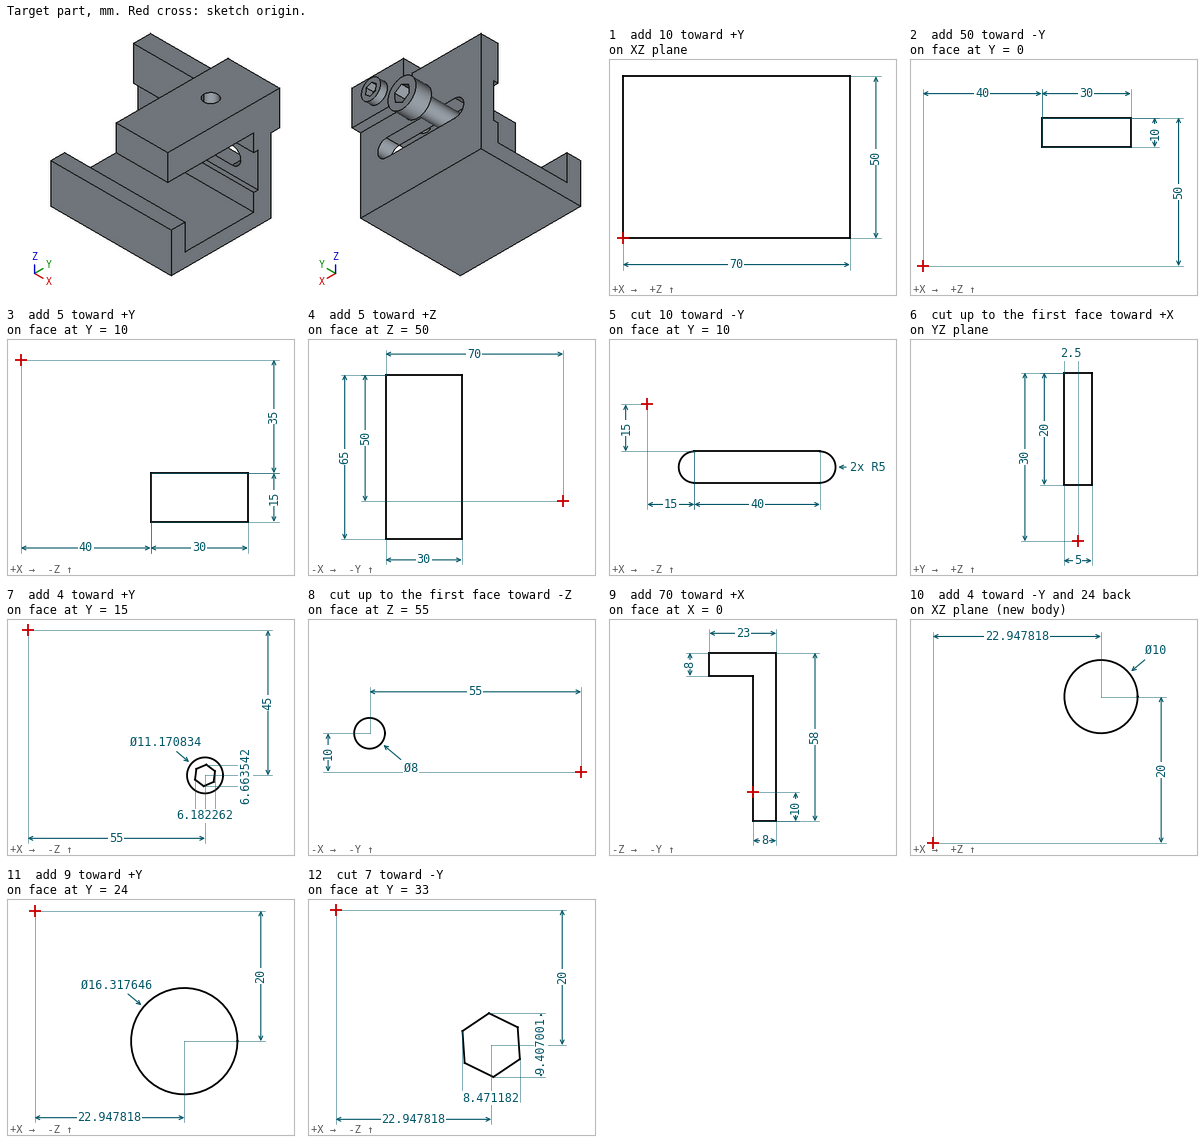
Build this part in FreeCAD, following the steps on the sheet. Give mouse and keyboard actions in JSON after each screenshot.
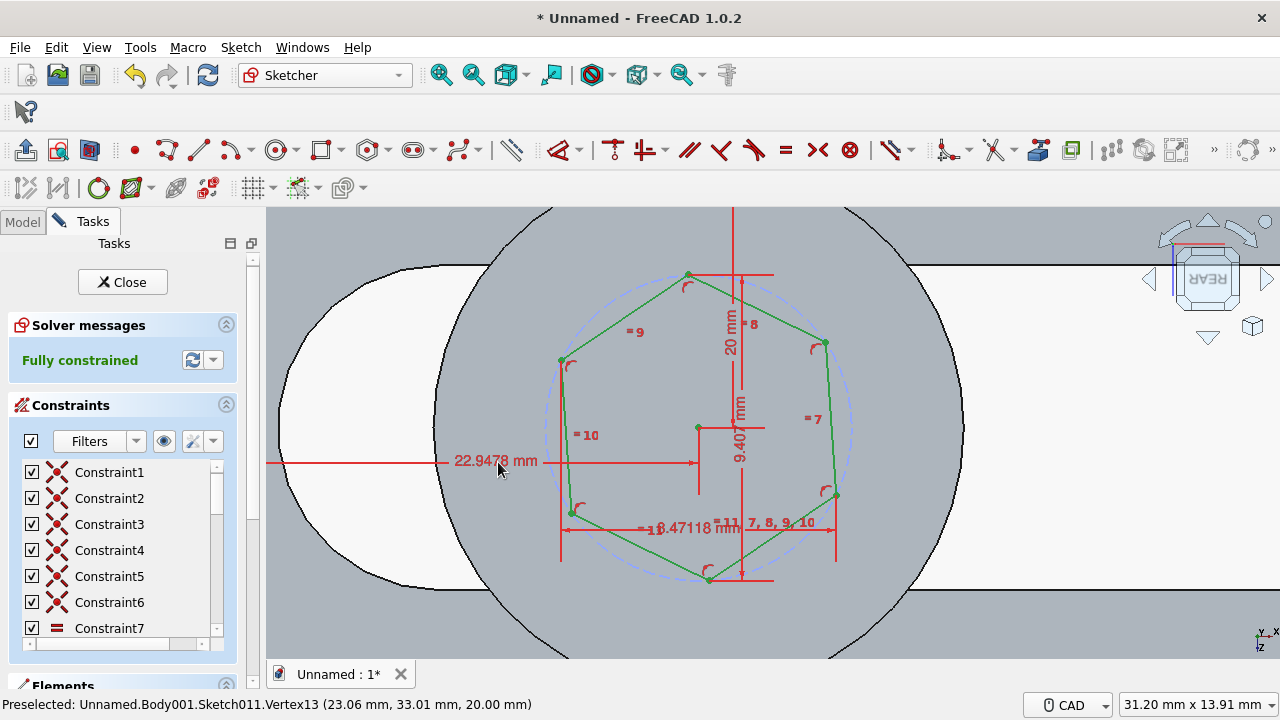
{"action": "left_click", "coordinate": [123, 282]}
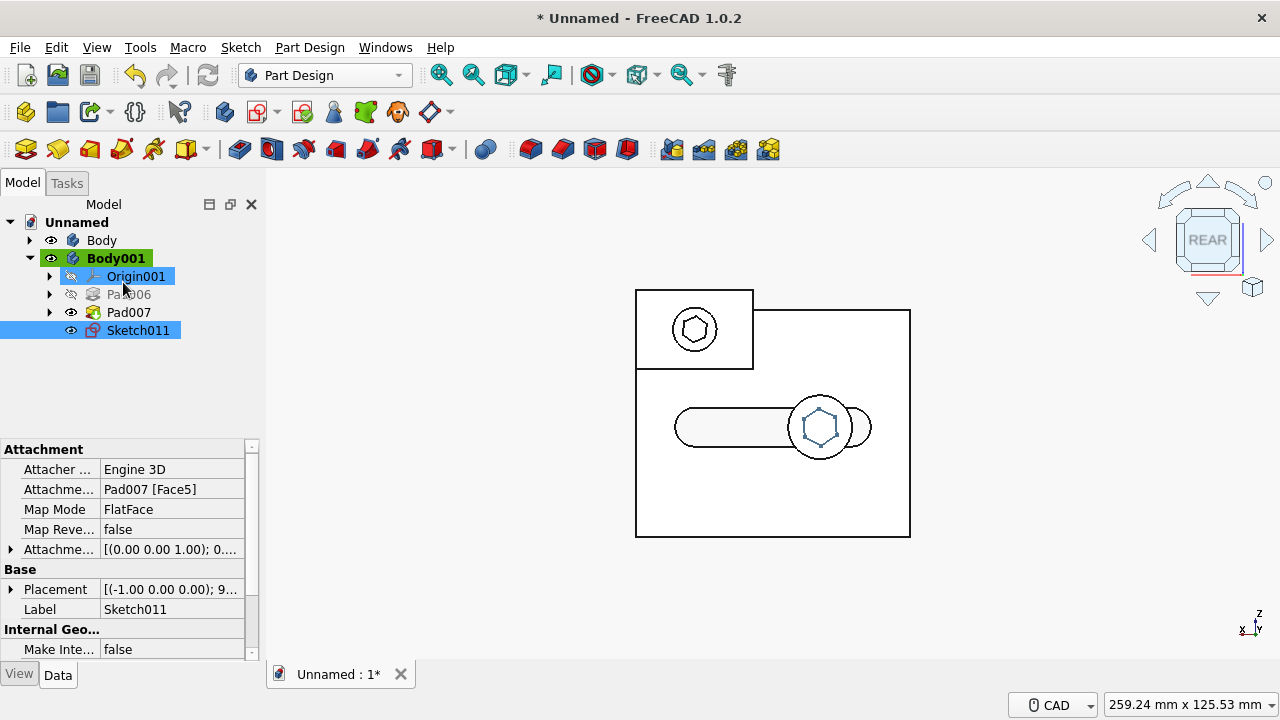
{"action": "left_click", "coordinate": [240, 150]}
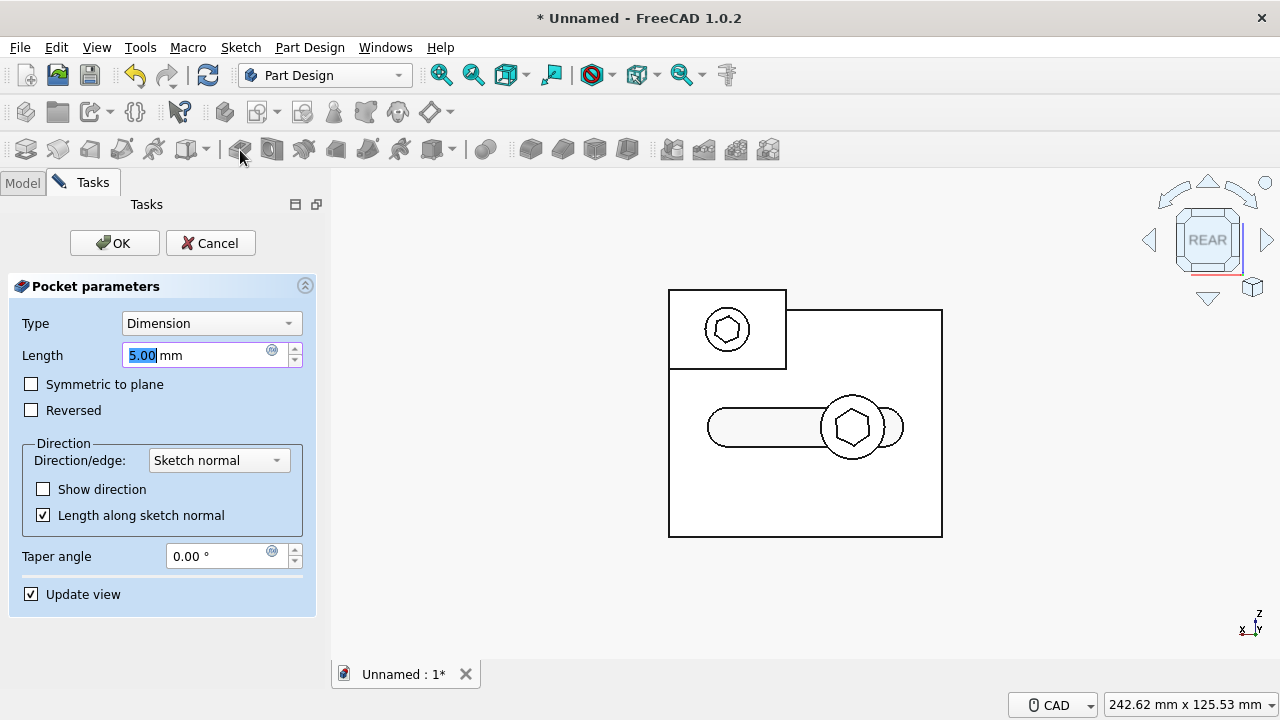
{"action": "type", "text": "7"}
{"action": "key", "text": "Tab"}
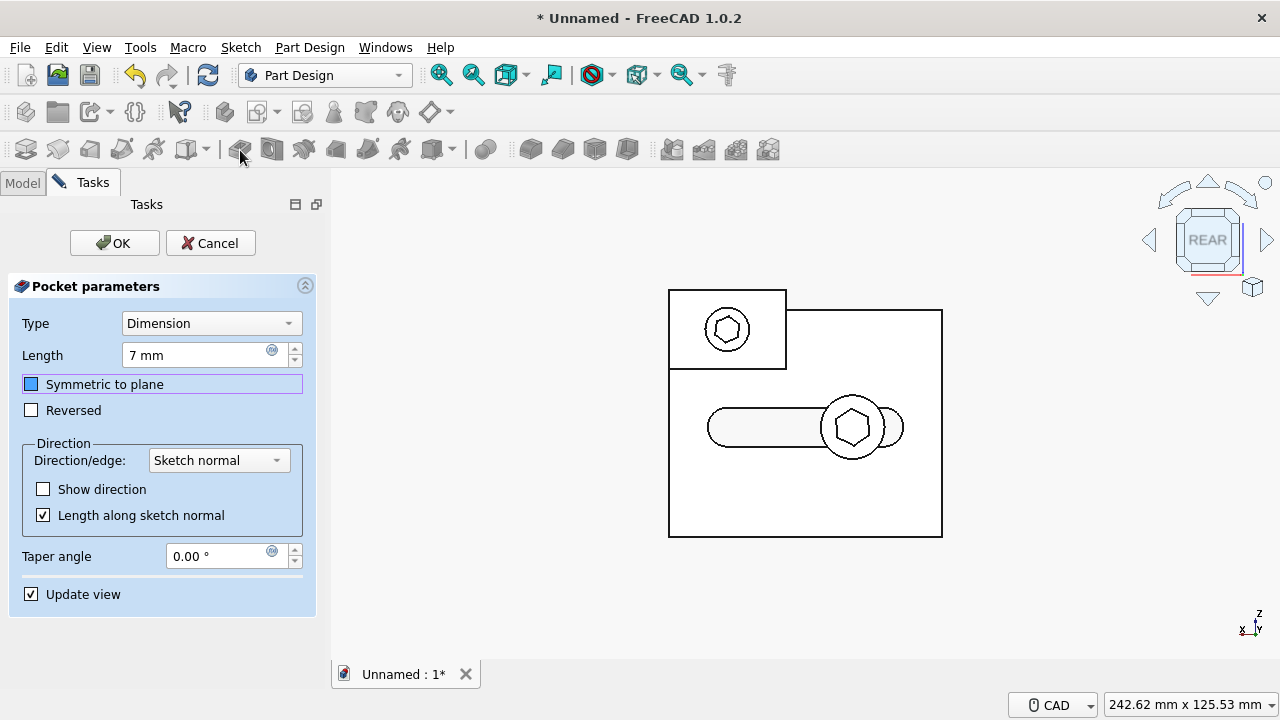
{"action": "left_click", "coordinate": [115, 243]}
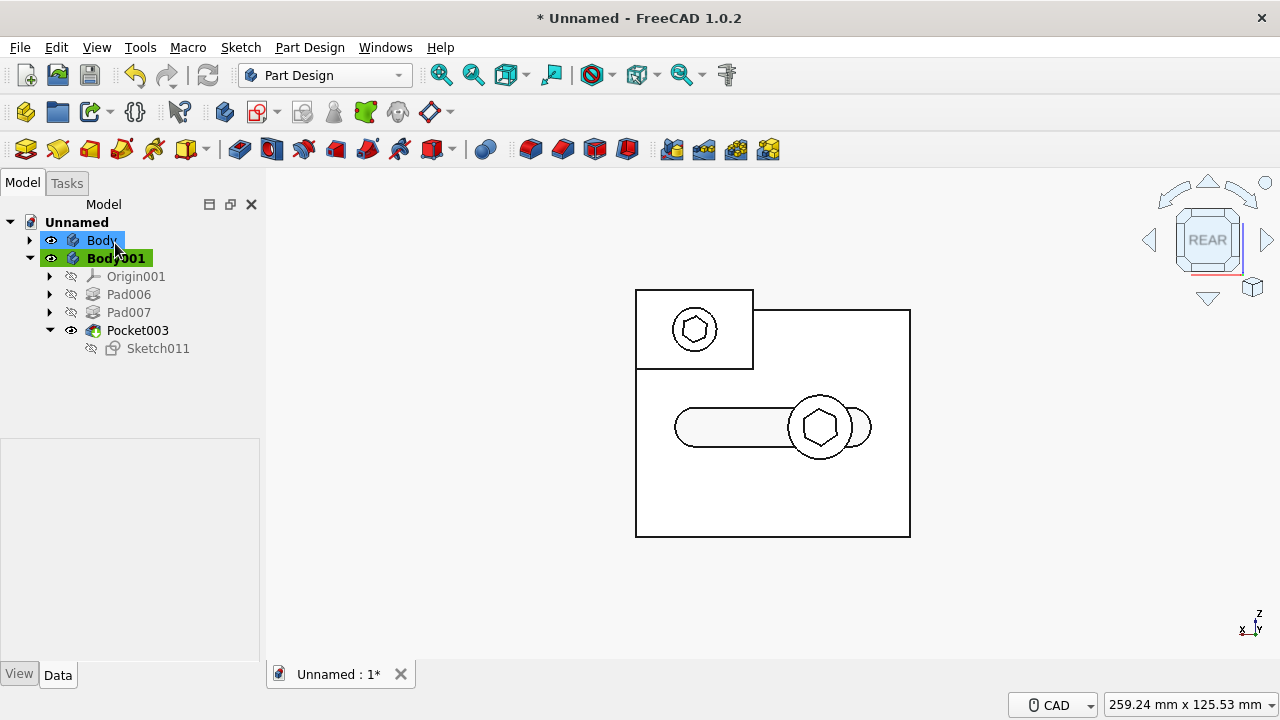
{"action": "key", "text": "0"}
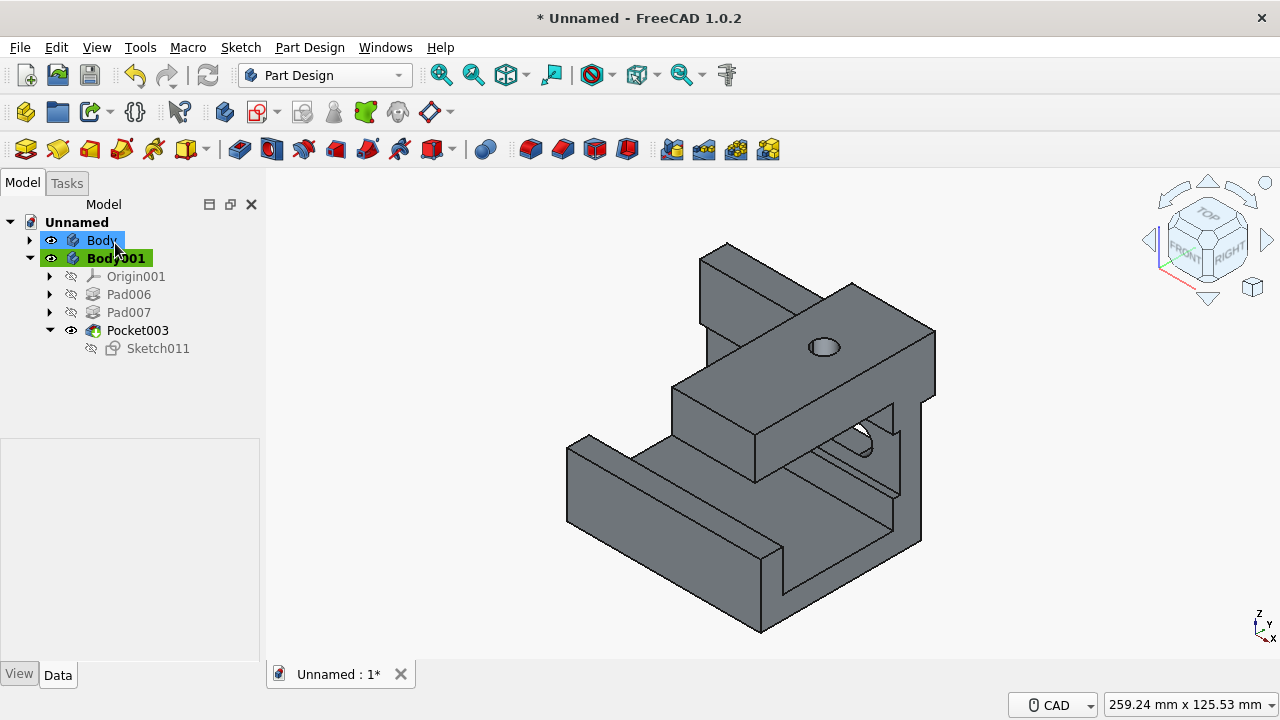
{"action": "left_click", "coordinate": [442, 76]}